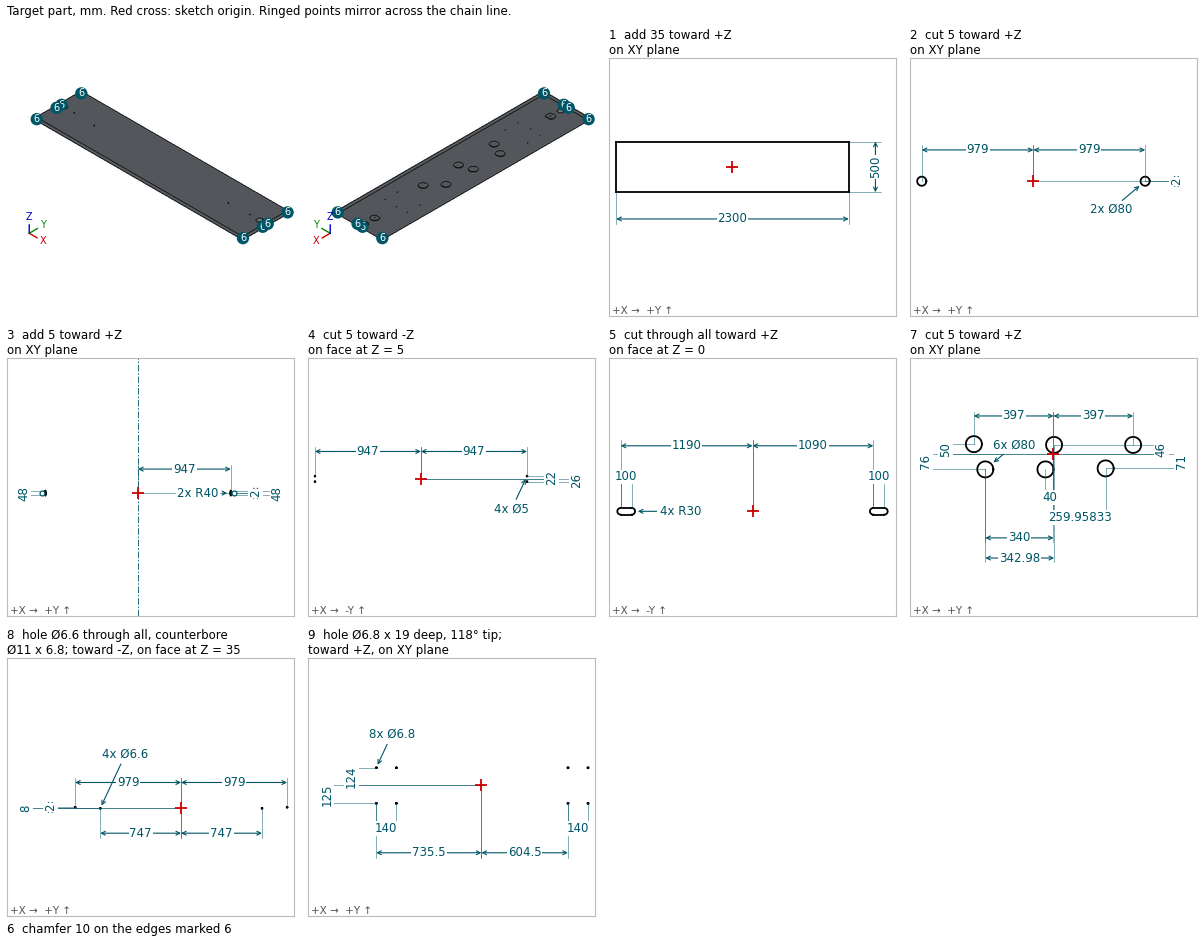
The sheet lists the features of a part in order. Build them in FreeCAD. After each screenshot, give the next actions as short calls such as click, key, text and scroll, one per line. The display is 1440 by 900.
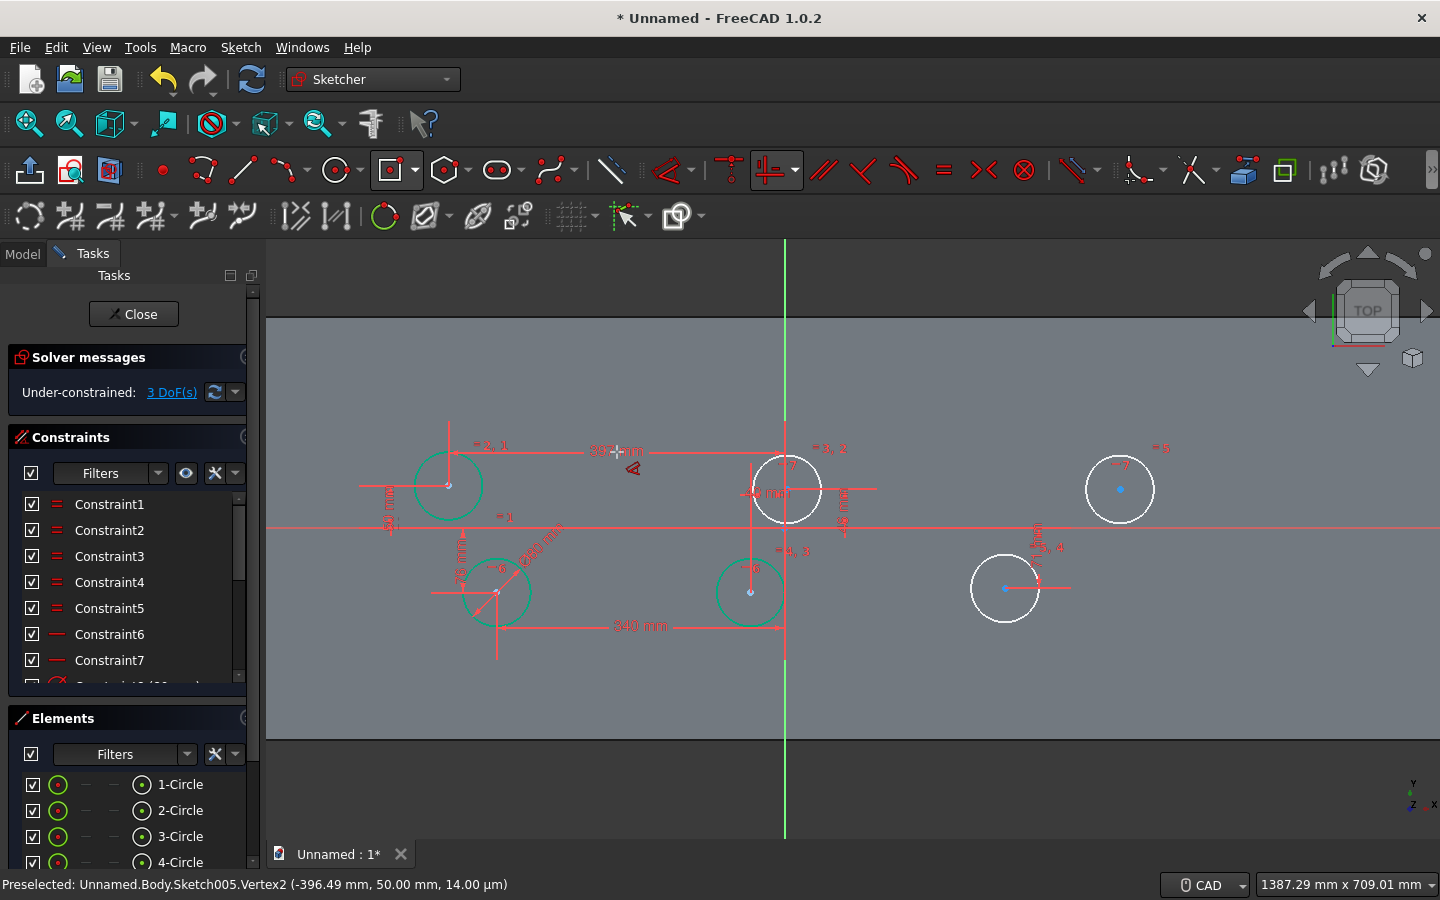
click(1120, 489)
click(952, 455)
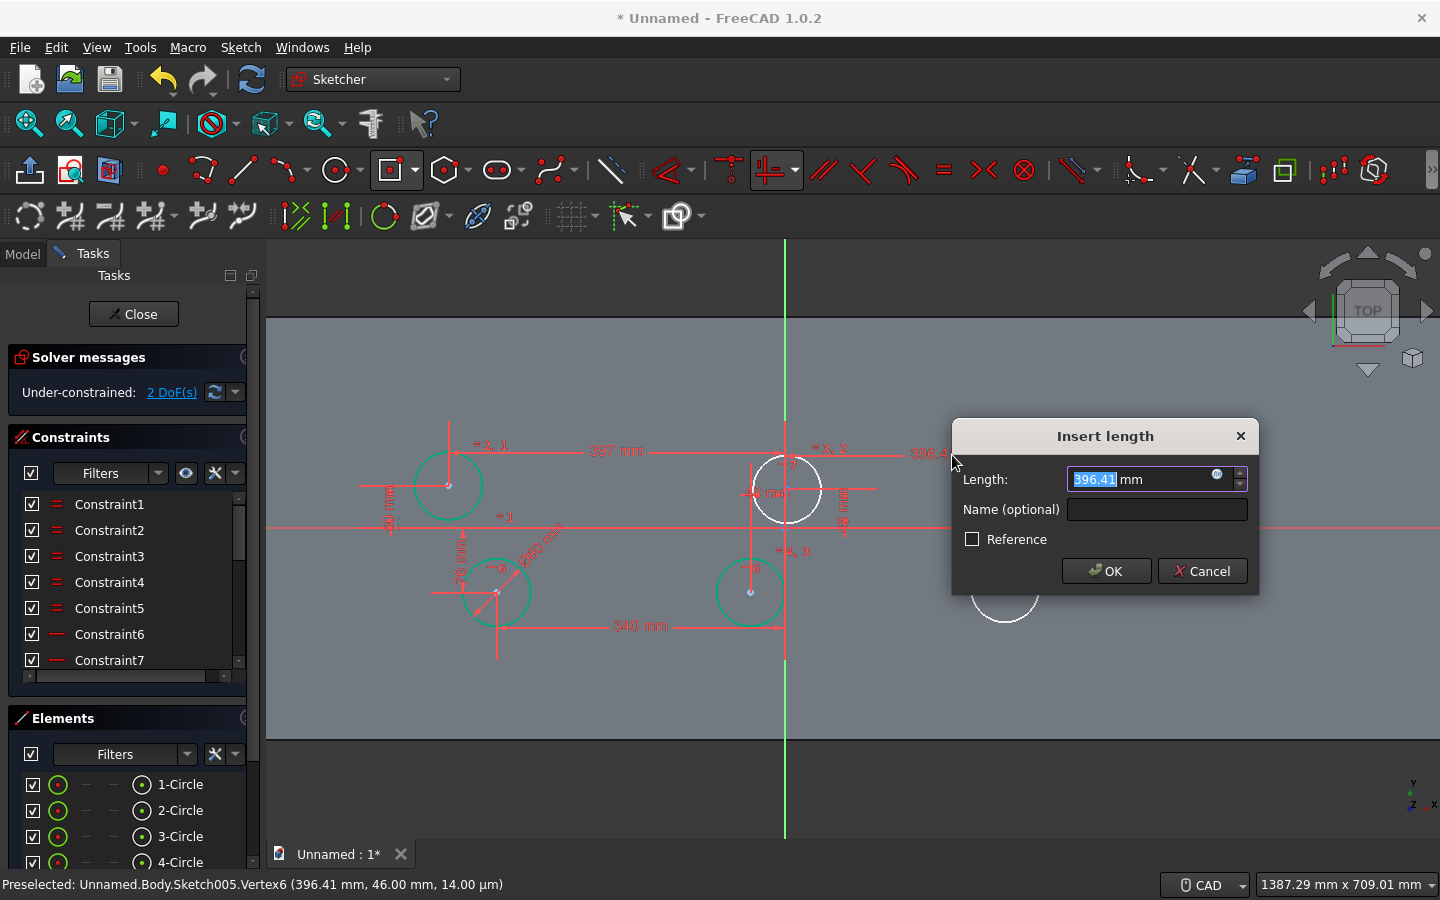
text(397)
key(Return)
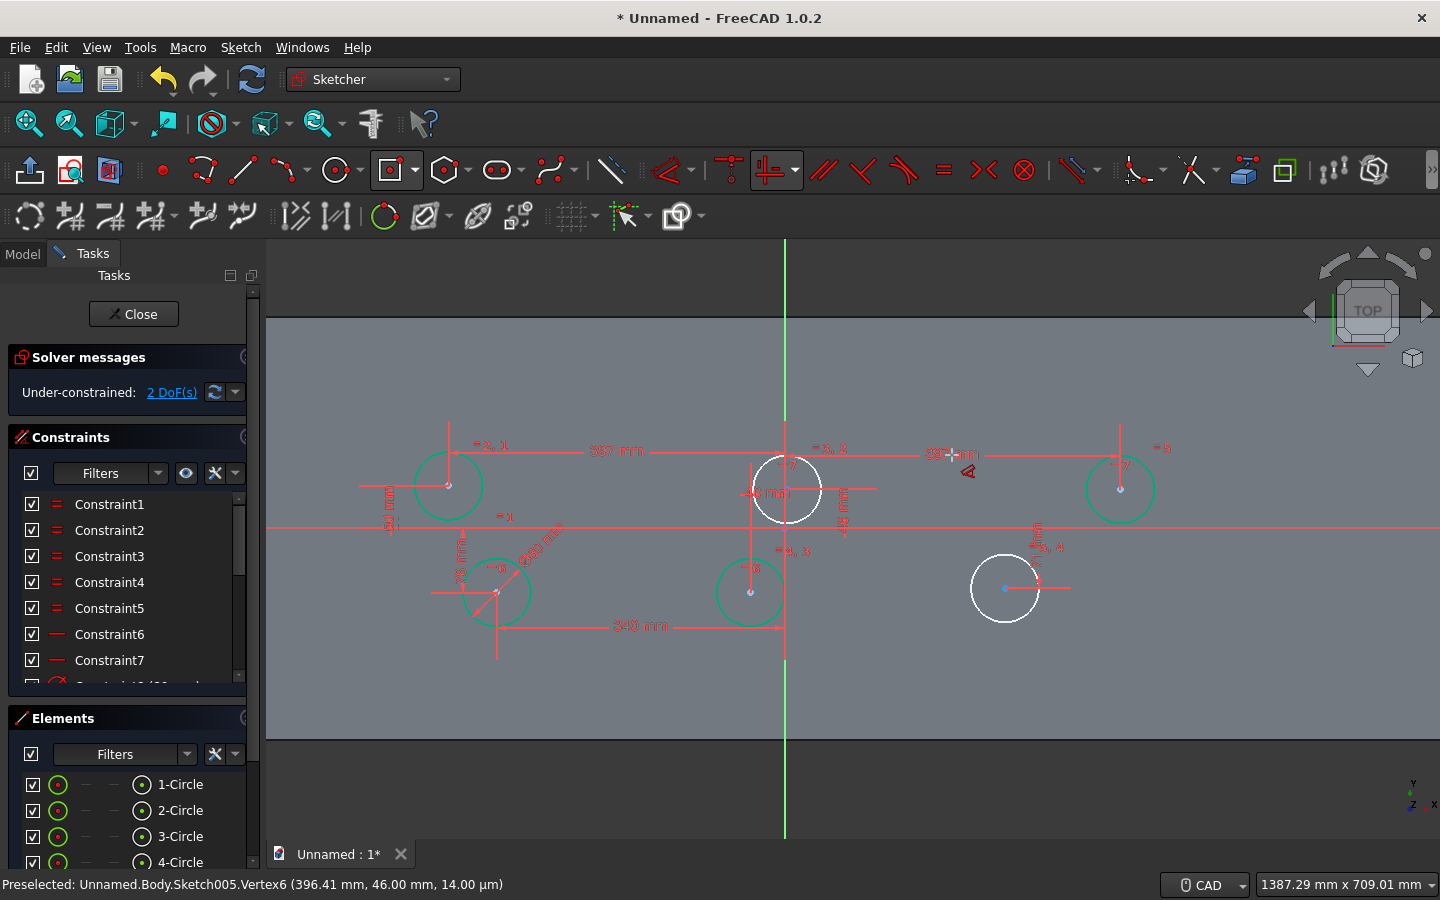
click(497, 593)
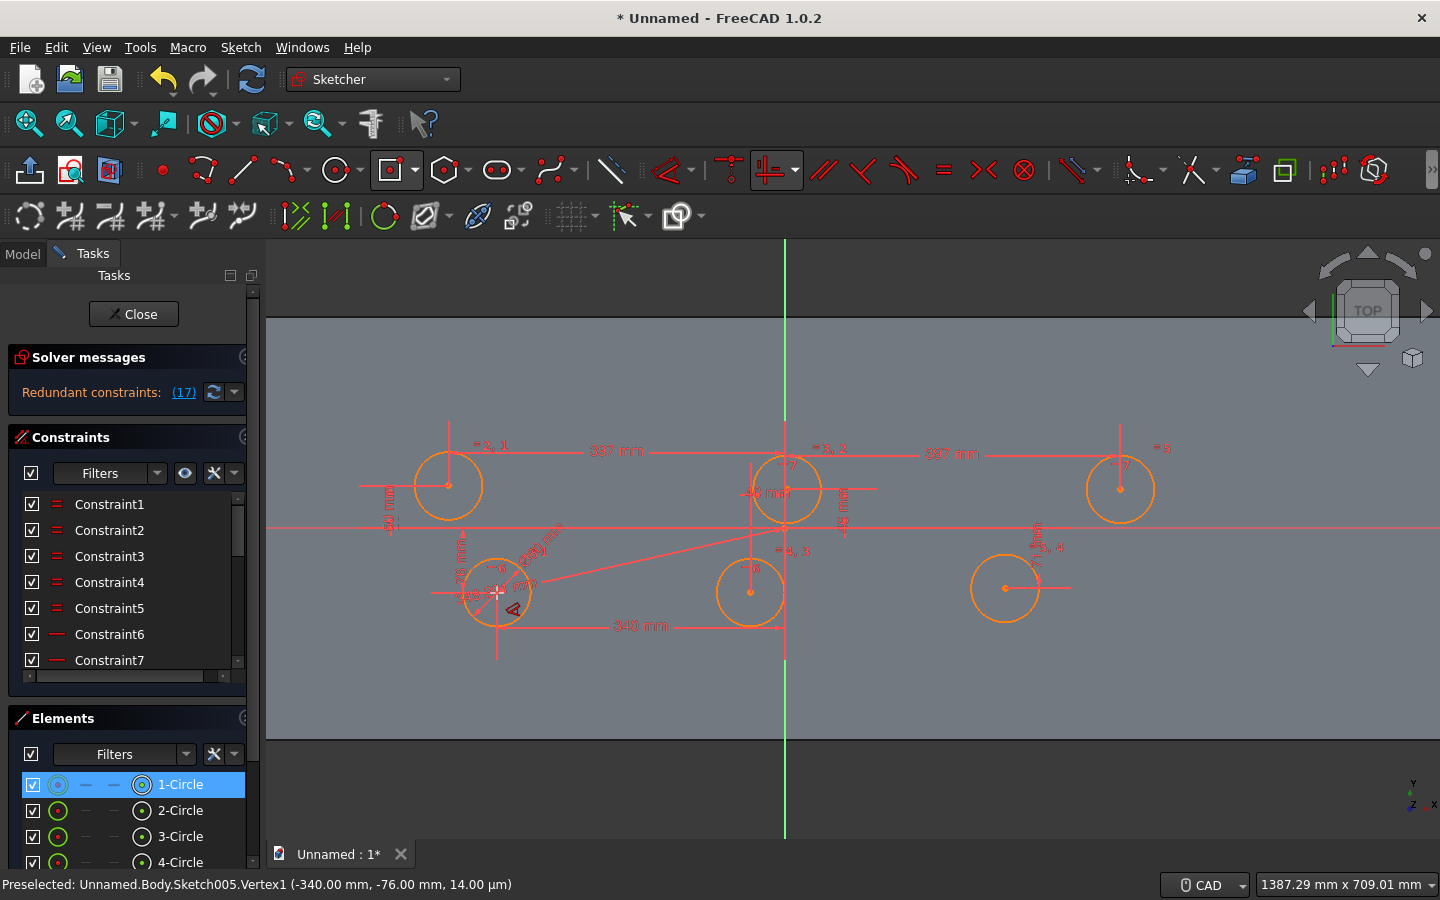
click(787, 489)
click(540, 627)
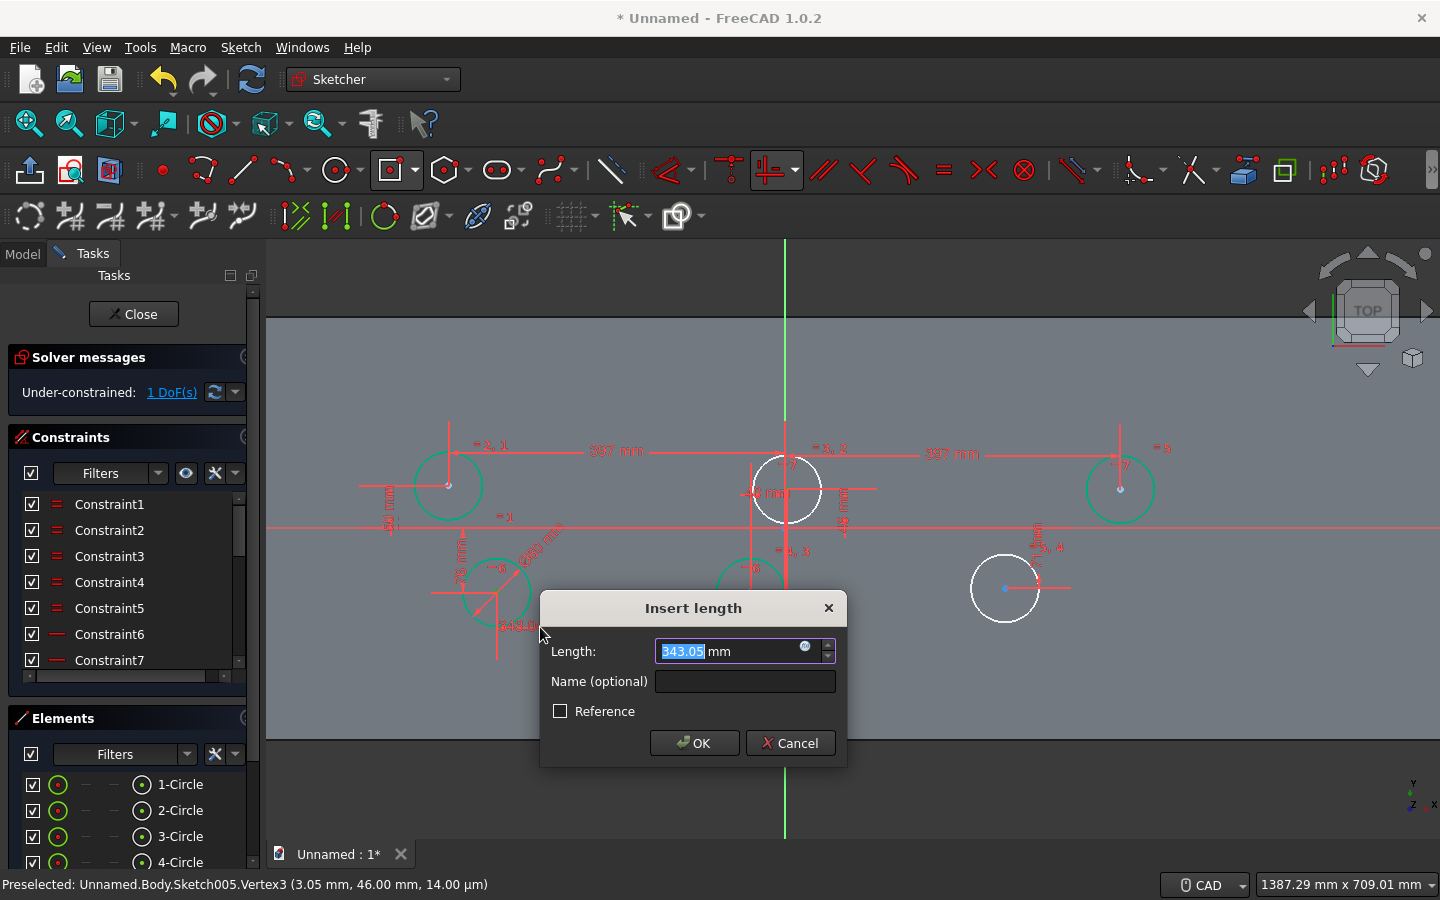
text(342.98)
key(Return)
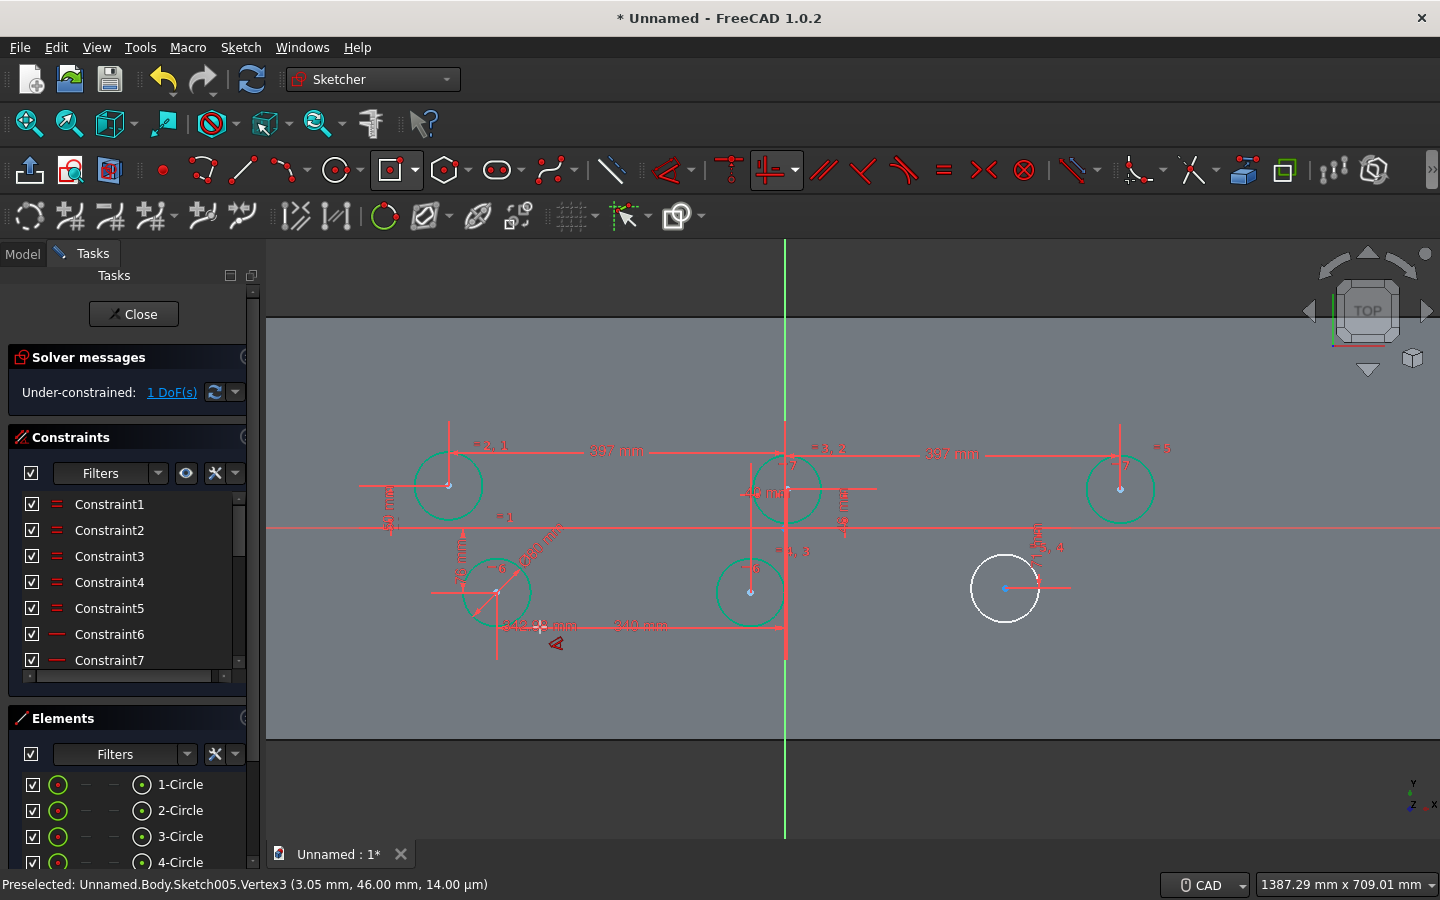
click(1005, 588)
click(895, 622)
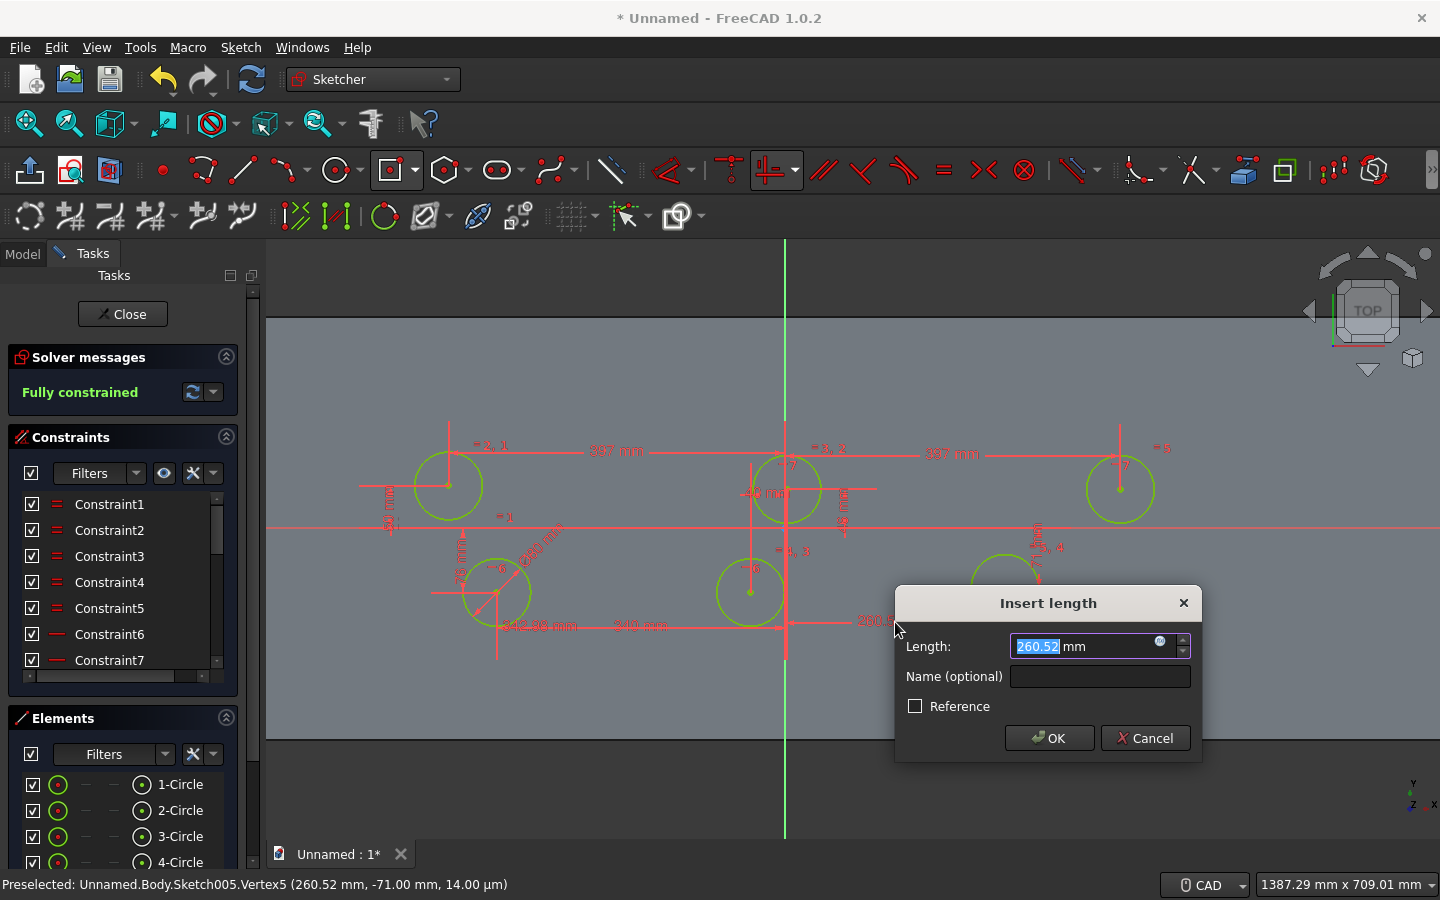
text(259.95833)
key(Return)
key(Escape)